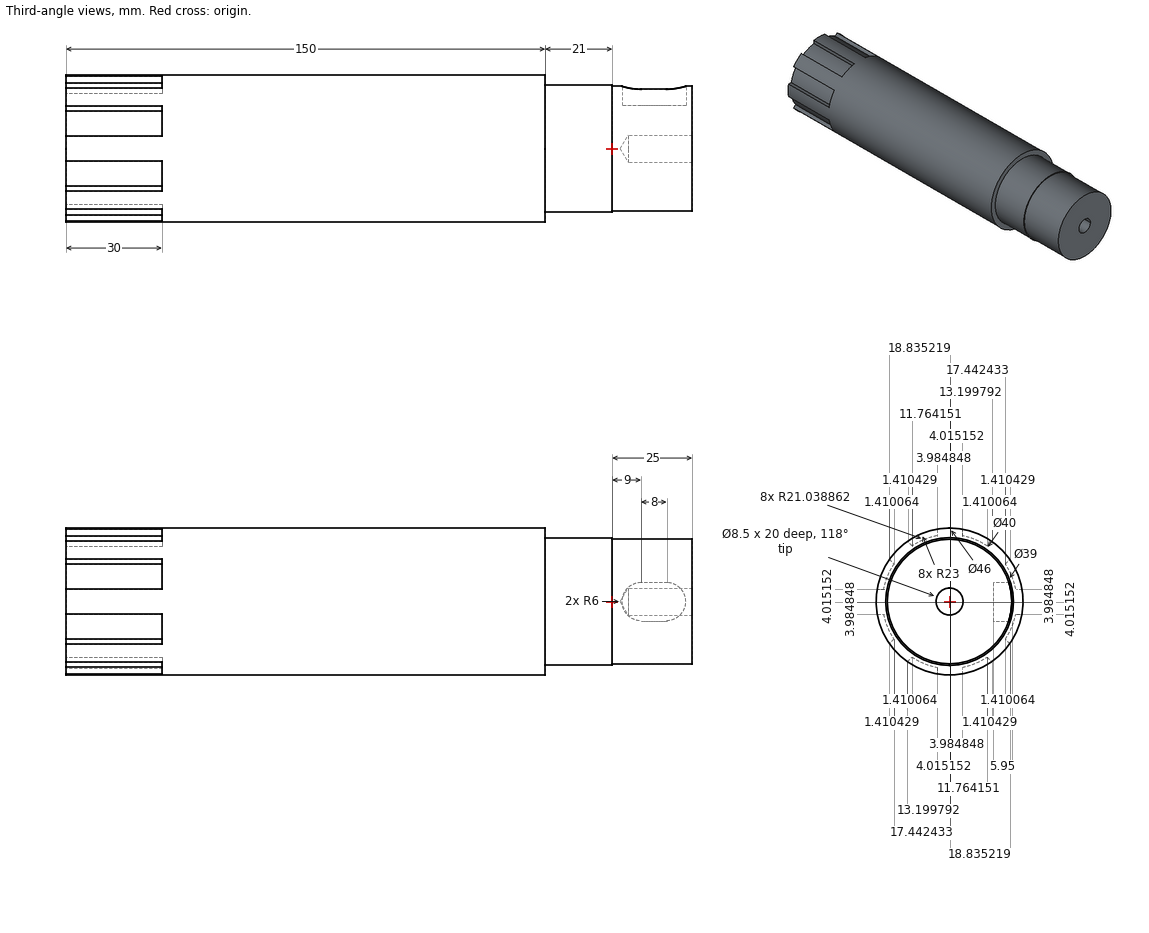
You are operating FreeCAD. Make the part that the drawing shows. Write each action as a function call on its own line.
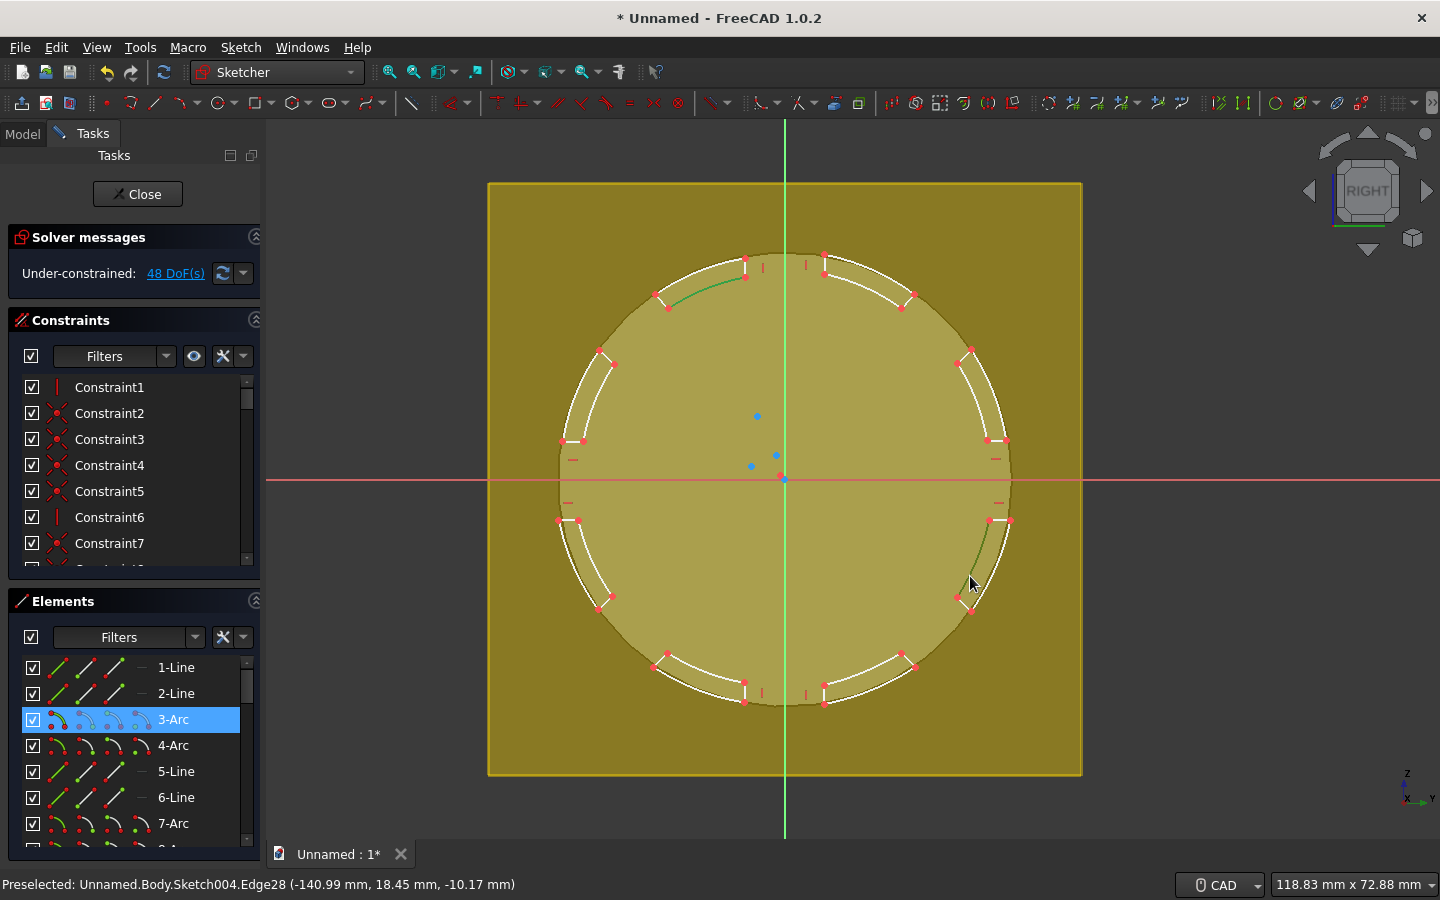
click(498, 104)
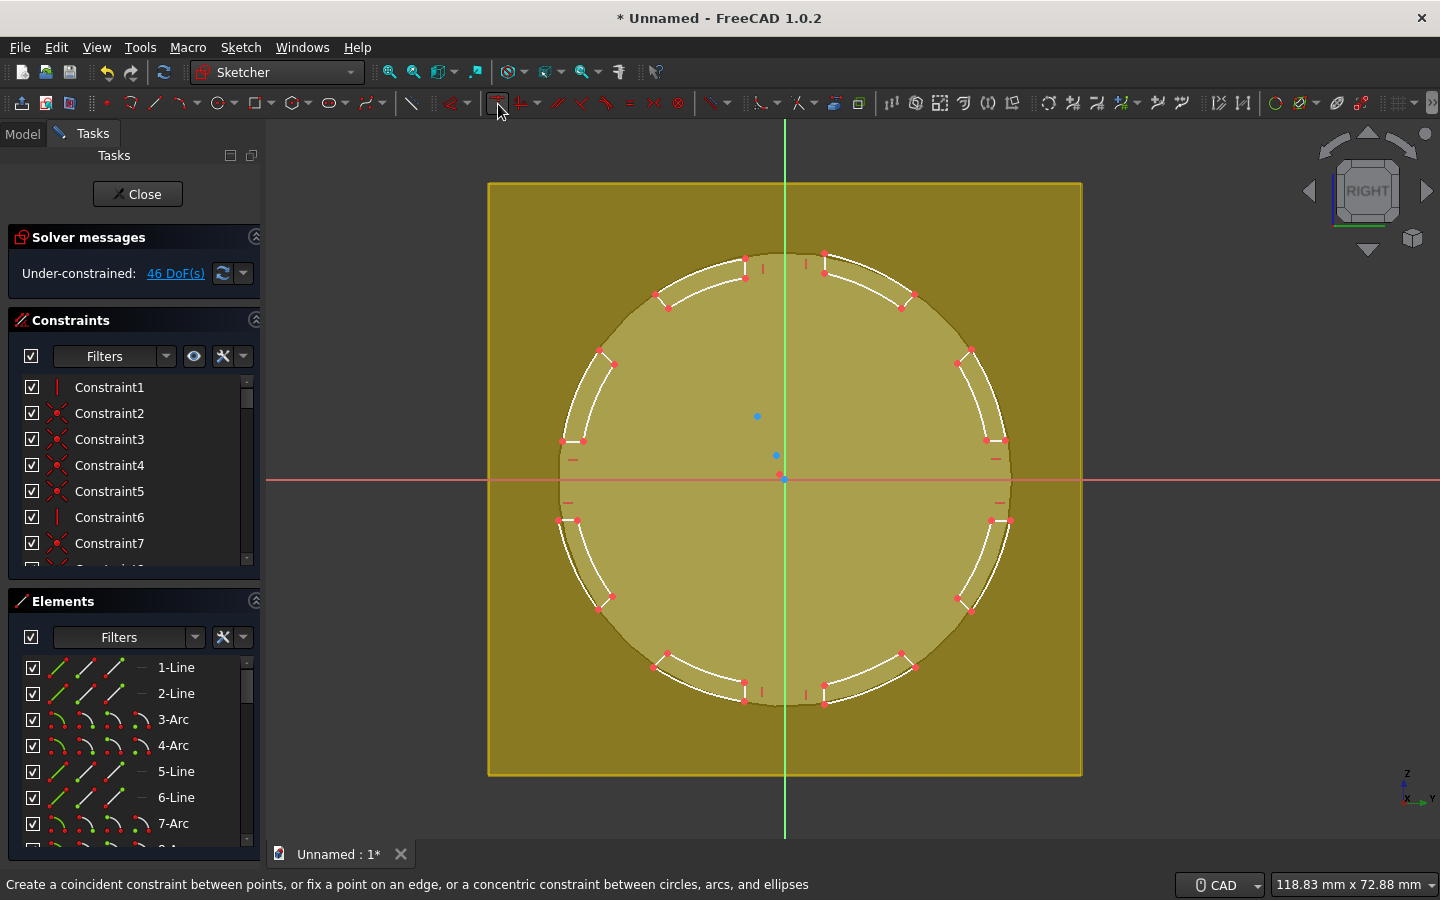
click(721, 284)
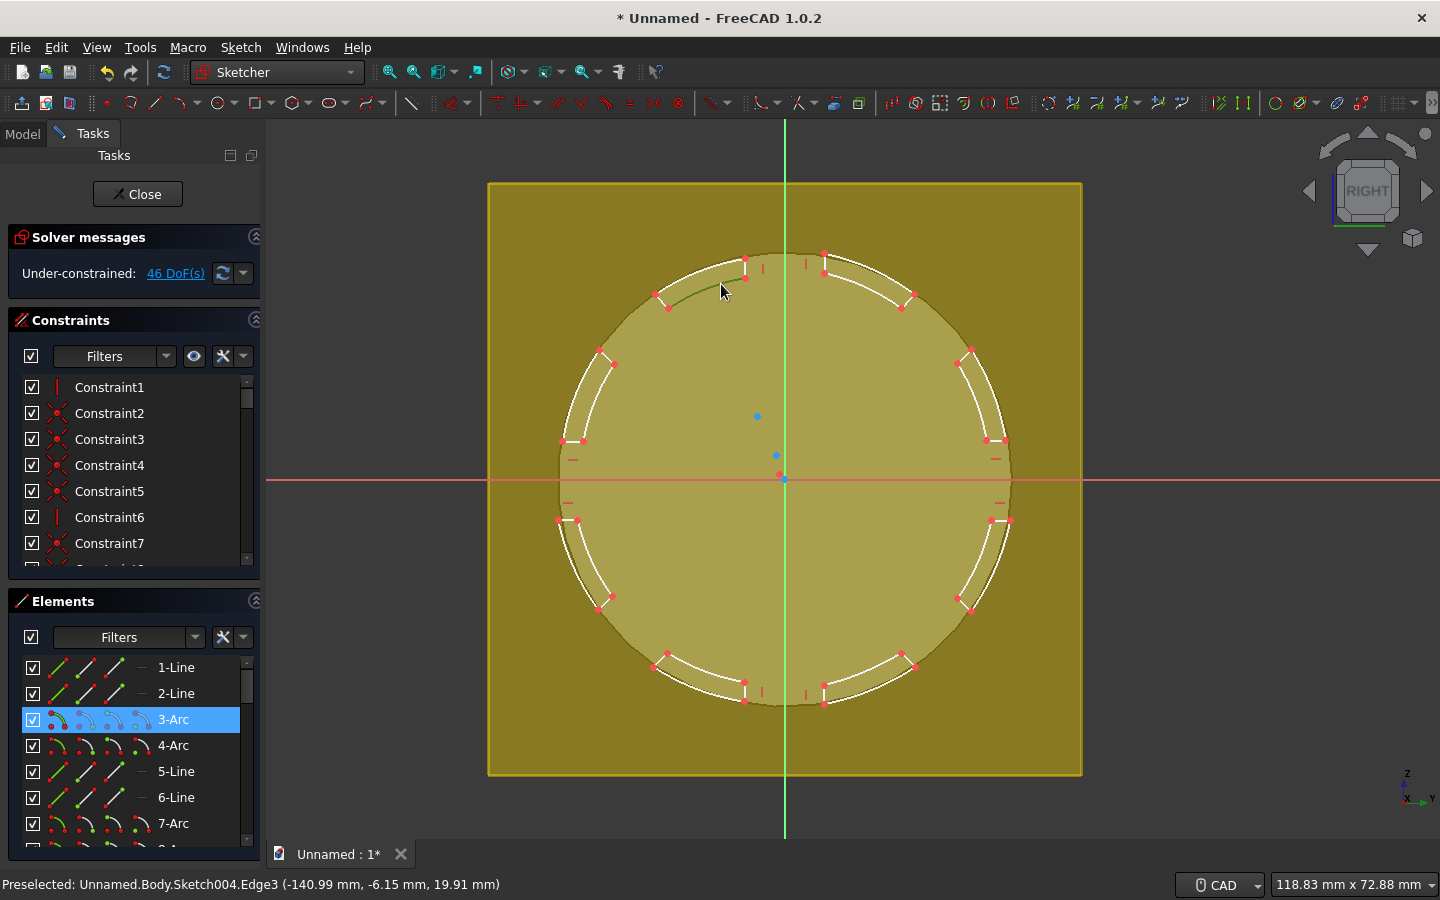
click(853, 697)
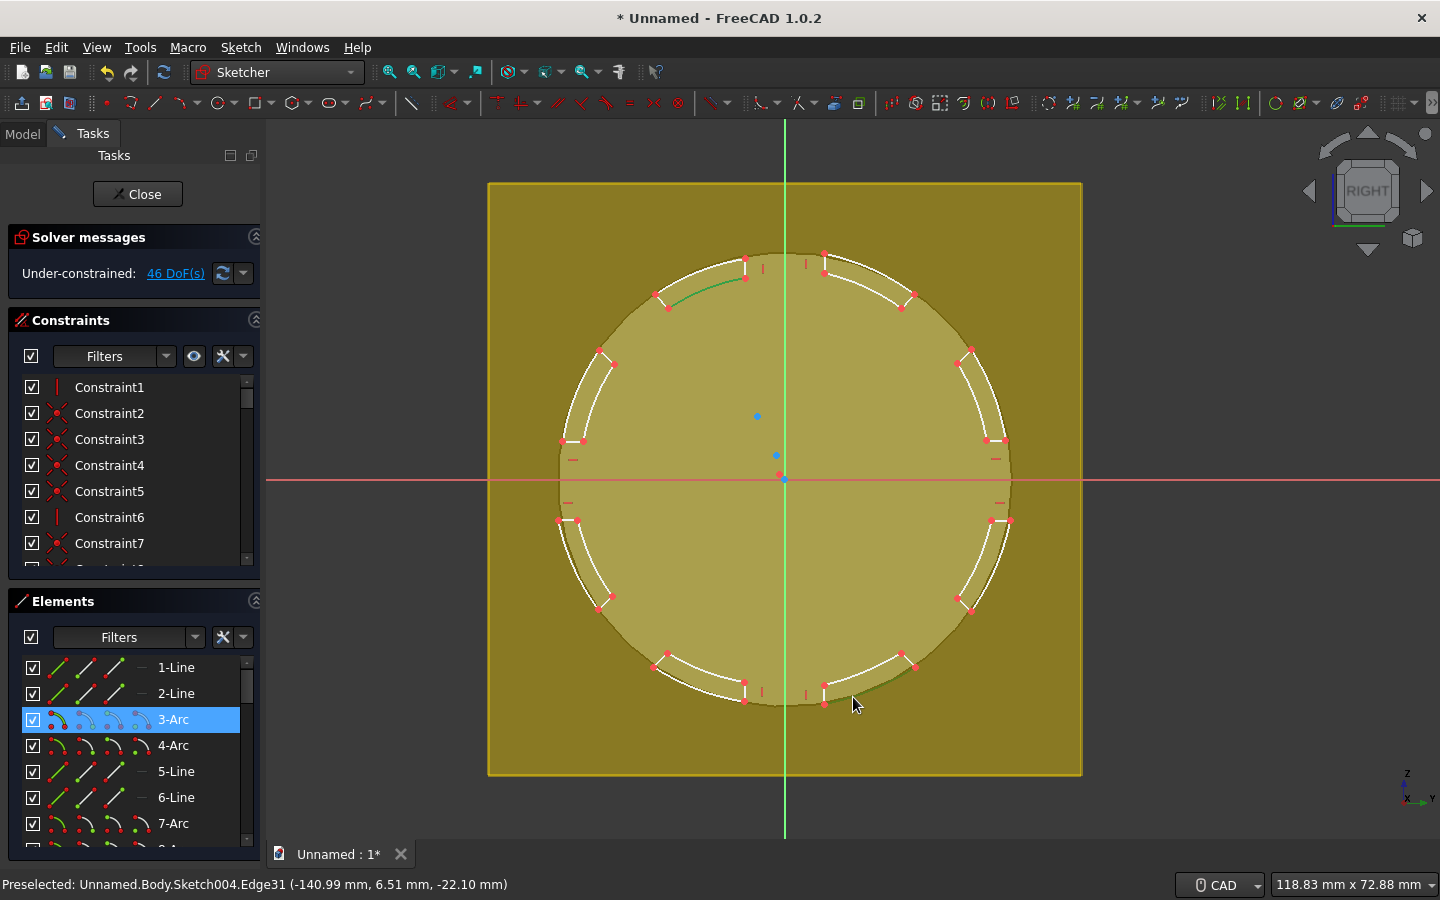
click(498, 104)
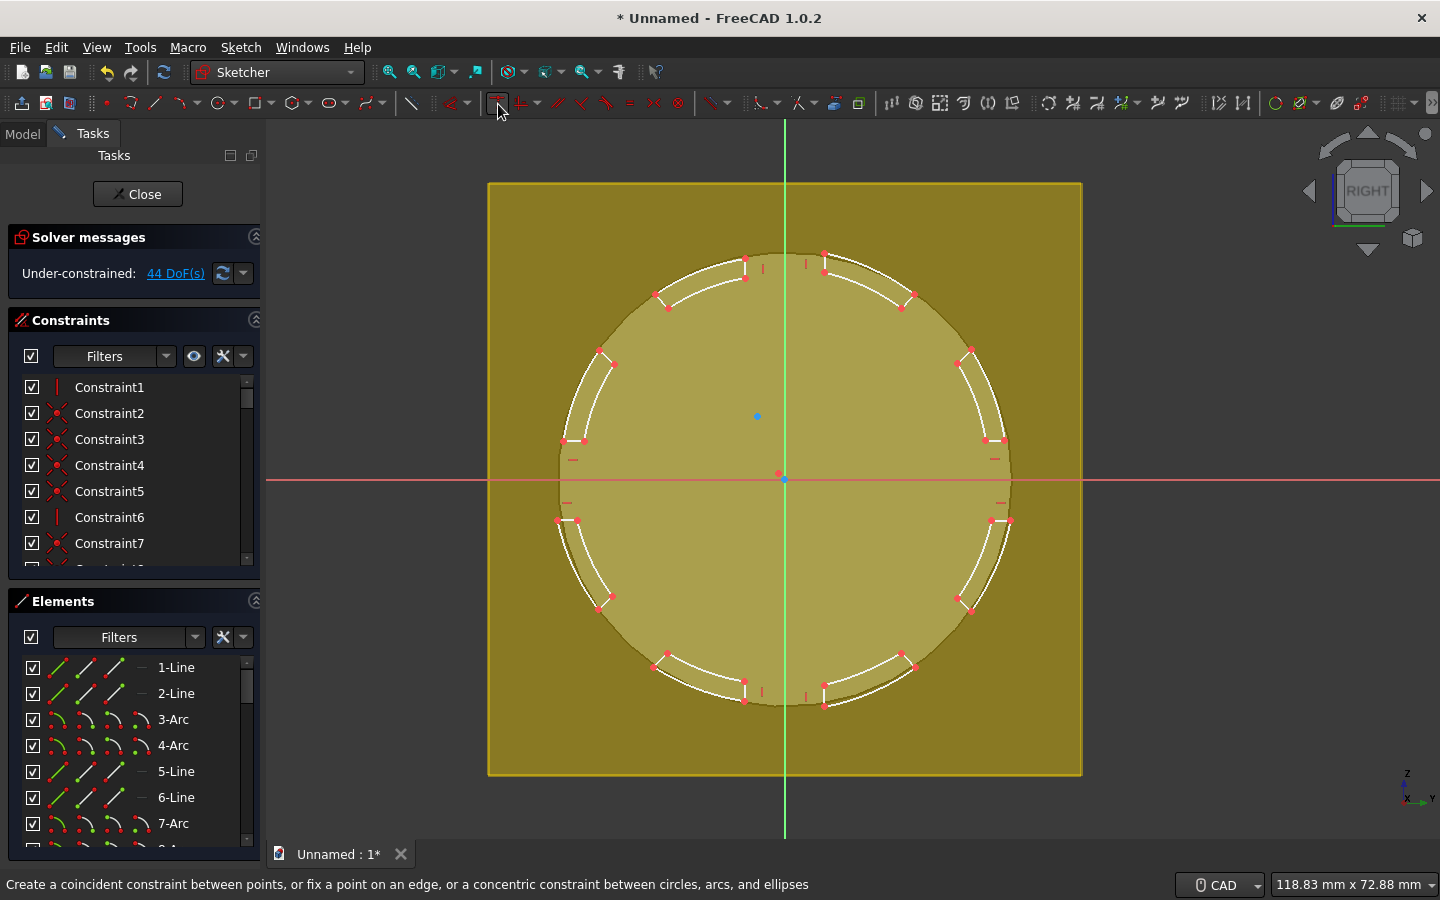
click(721, 284)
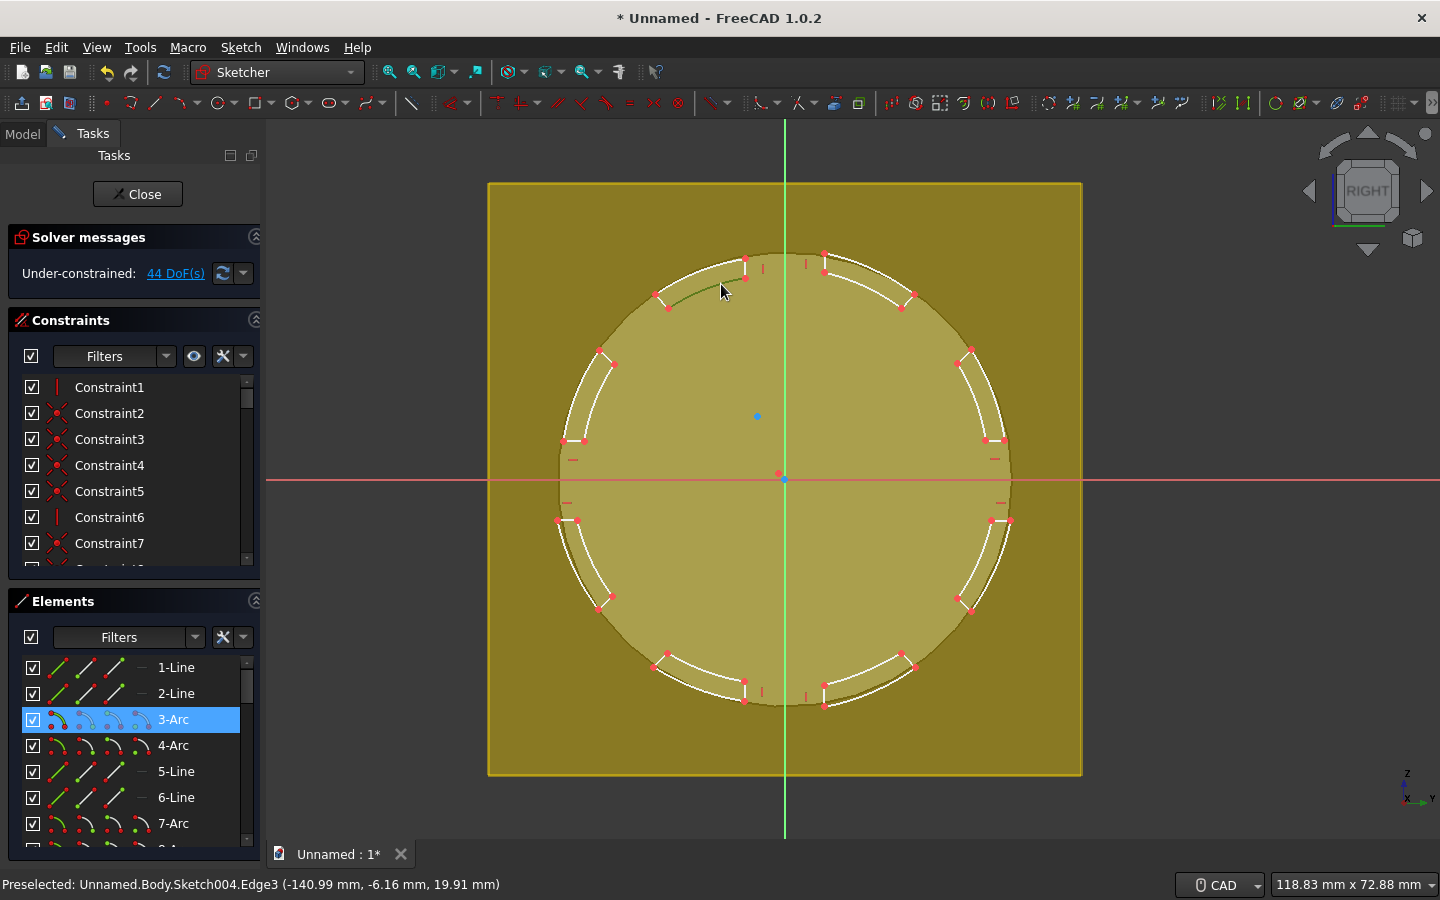
click(848, 678)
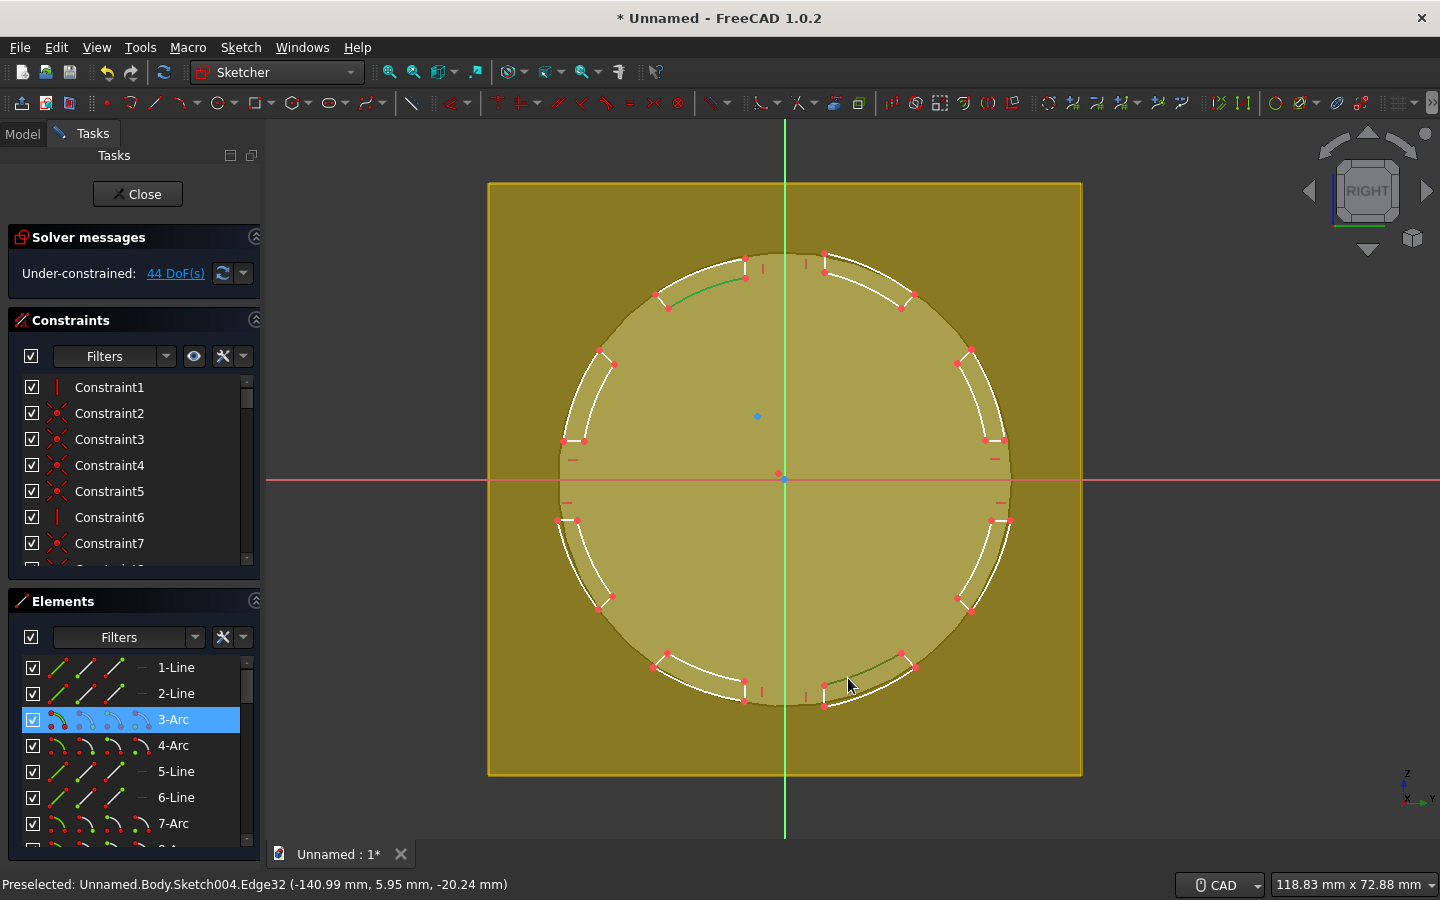
click(498, 104)